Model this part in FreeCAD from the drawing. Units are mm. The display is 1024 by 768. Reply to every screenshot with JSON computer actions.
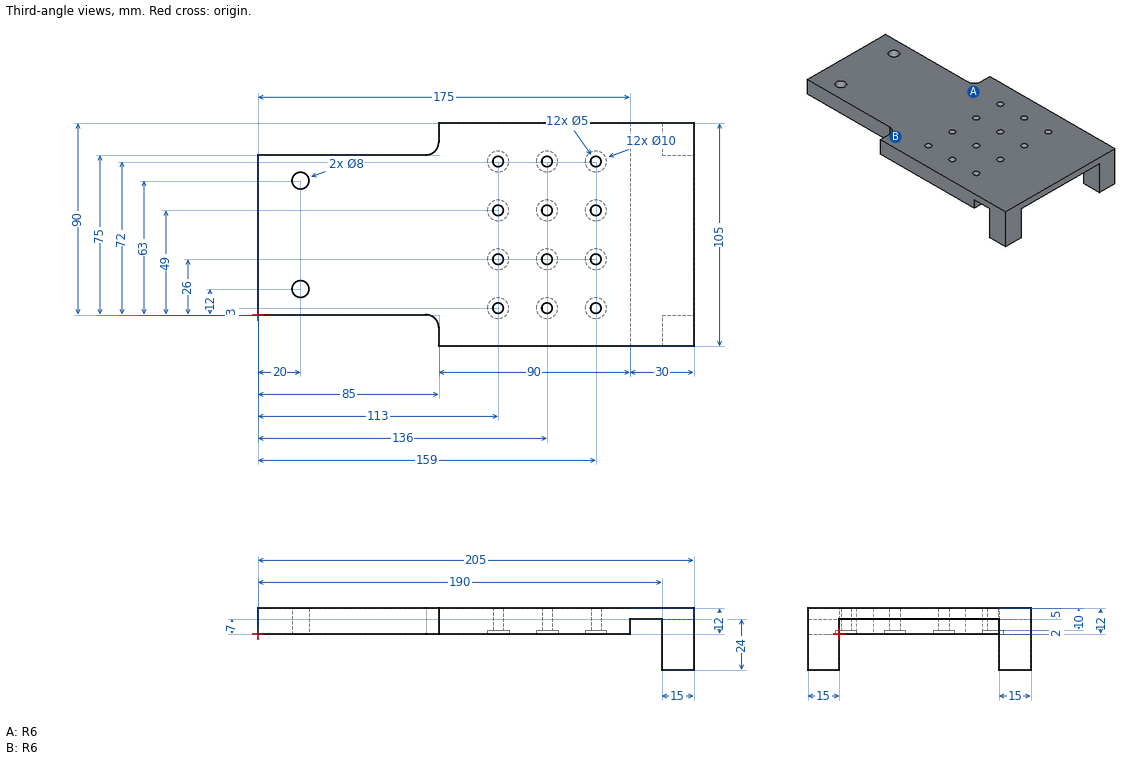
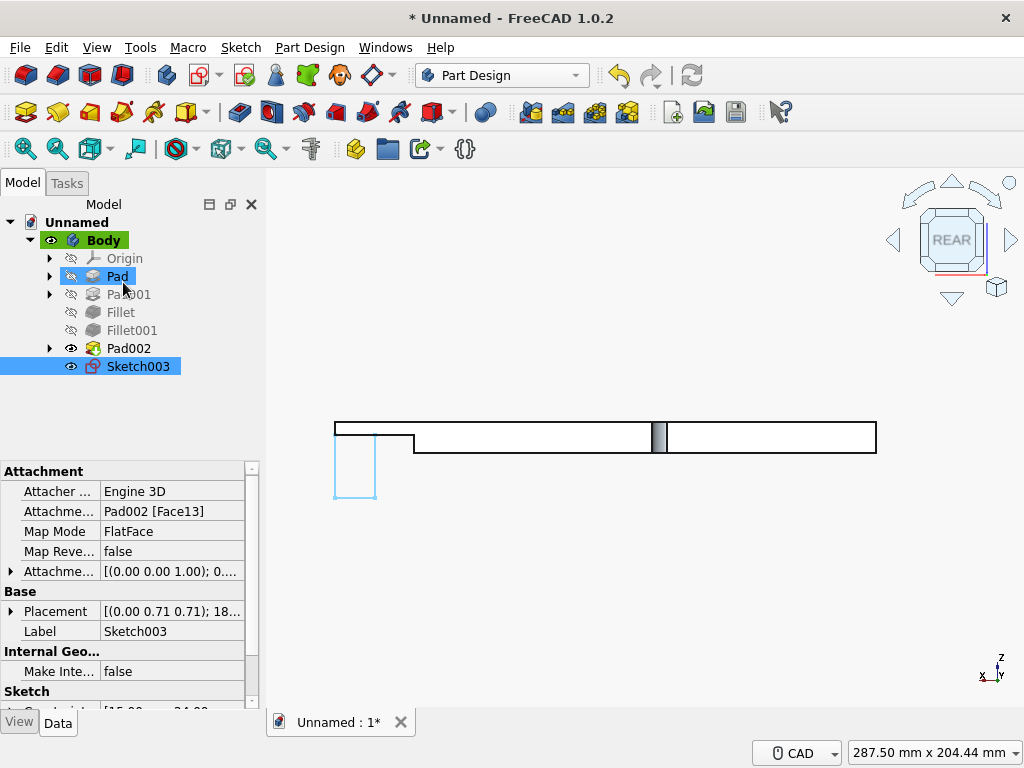
{"action": "left_click", "coordinate": [26, 112]}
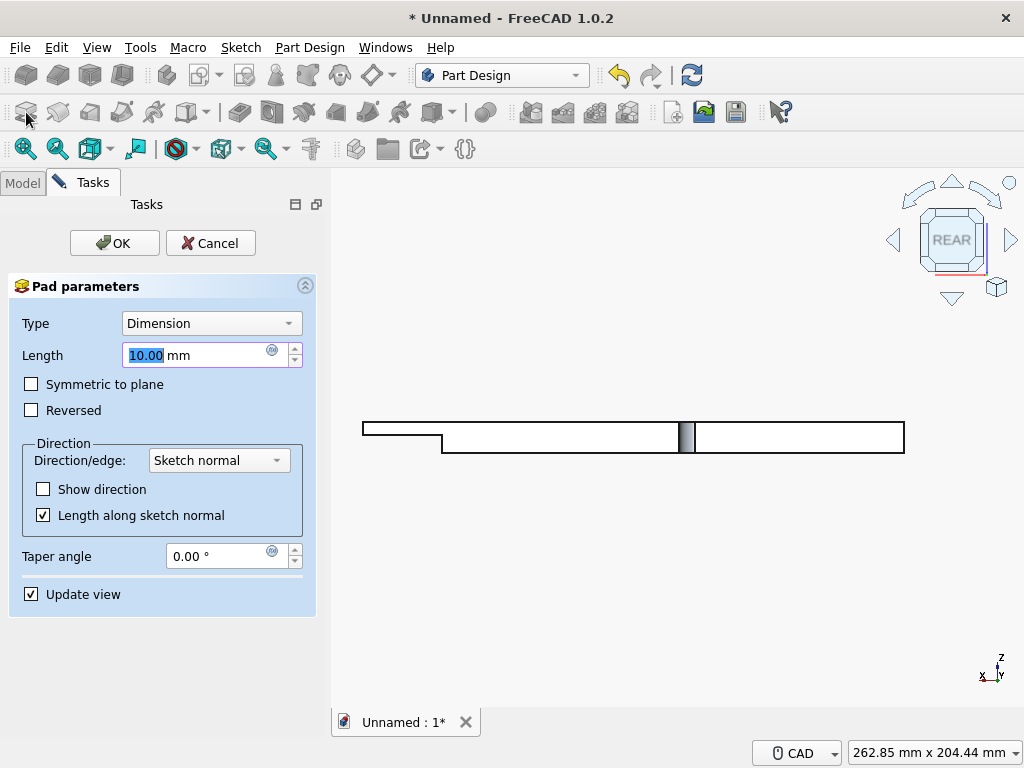
{"action": "type", "text": "15"}
{"action": "key", "text": "Tab"}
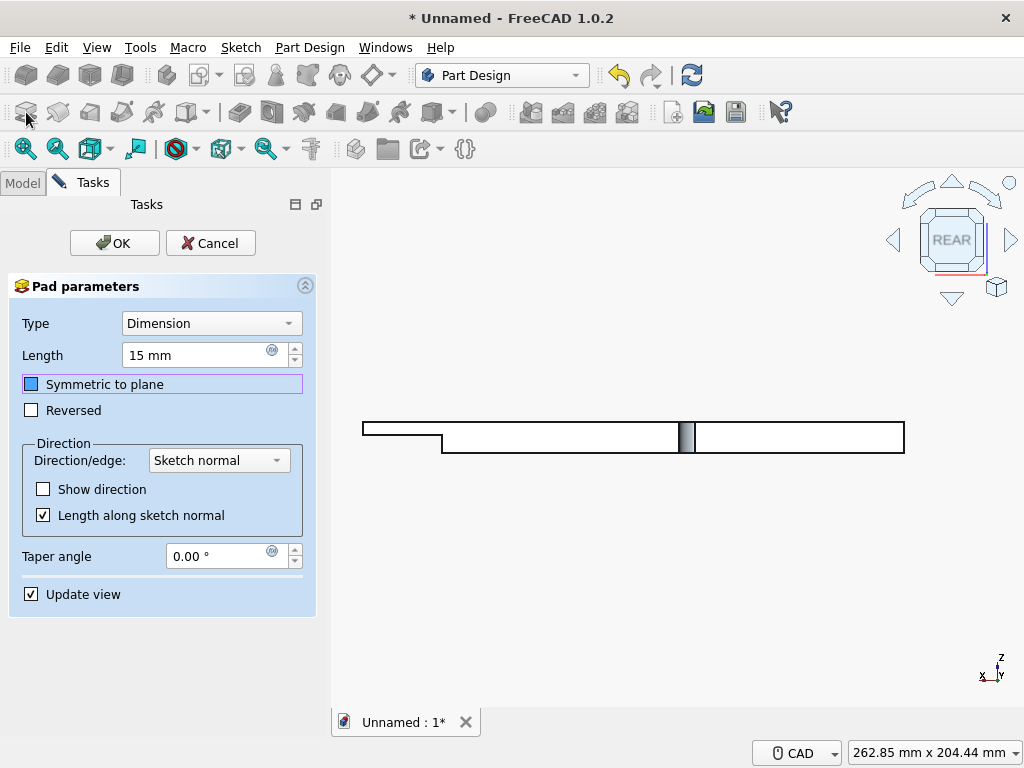
{"action": "left_click", "coordinate": [30, 410]}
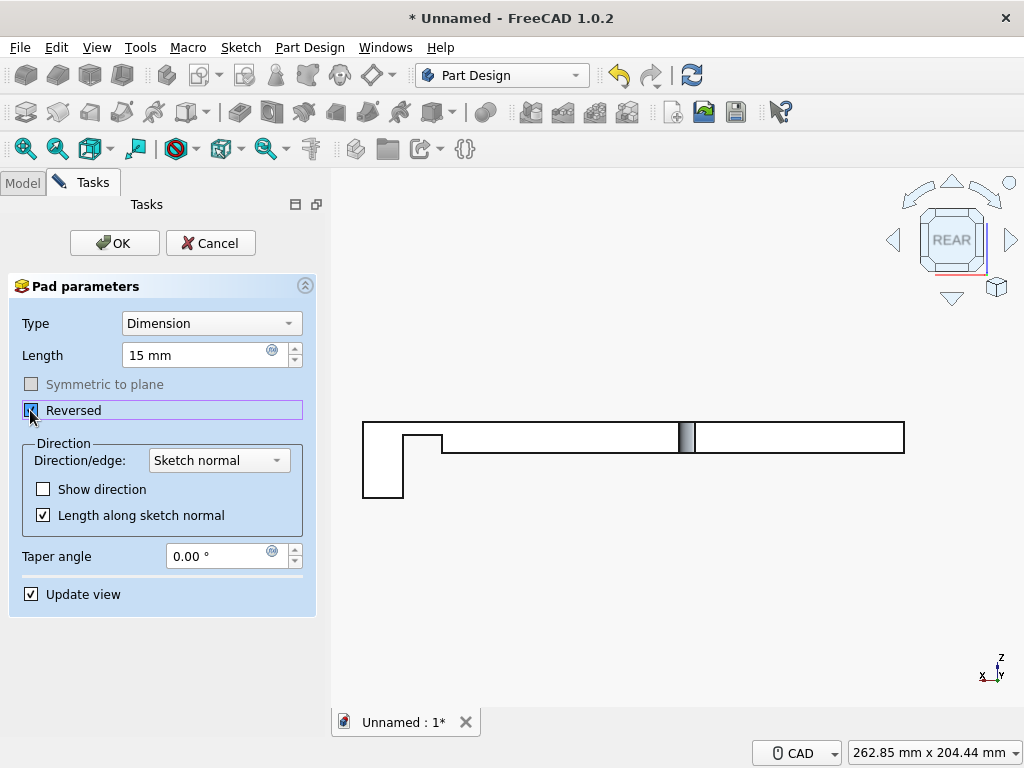
{"action": "left_click", "coordinate": [115, 243]}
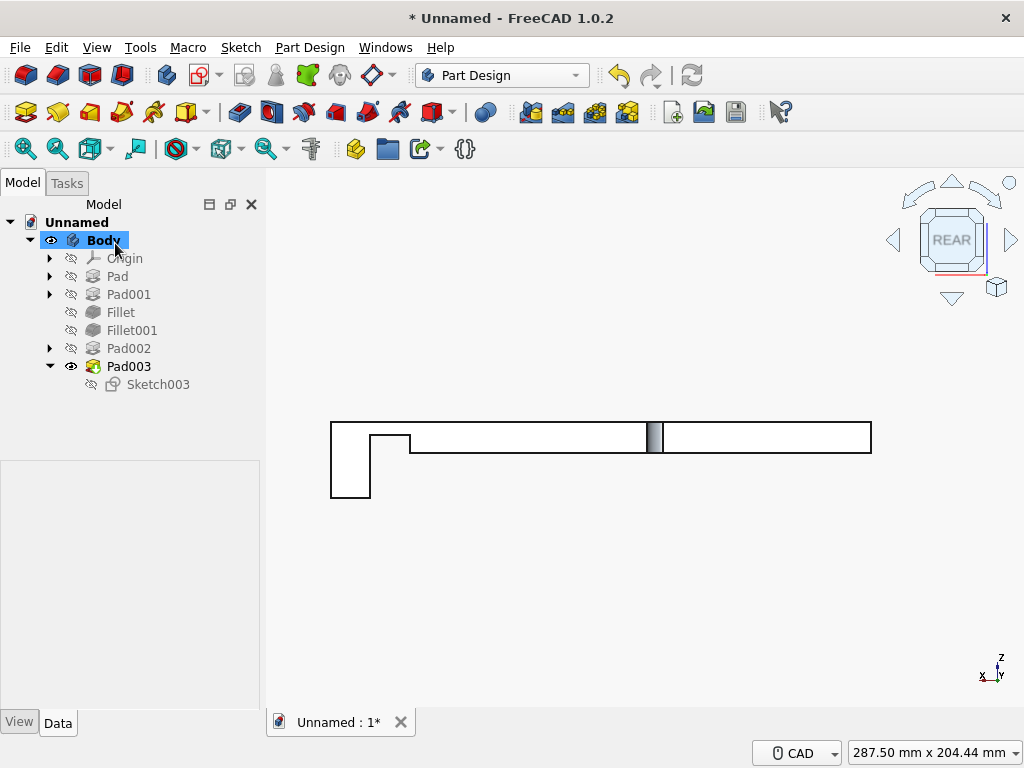
{"action": "key", "text": "0"}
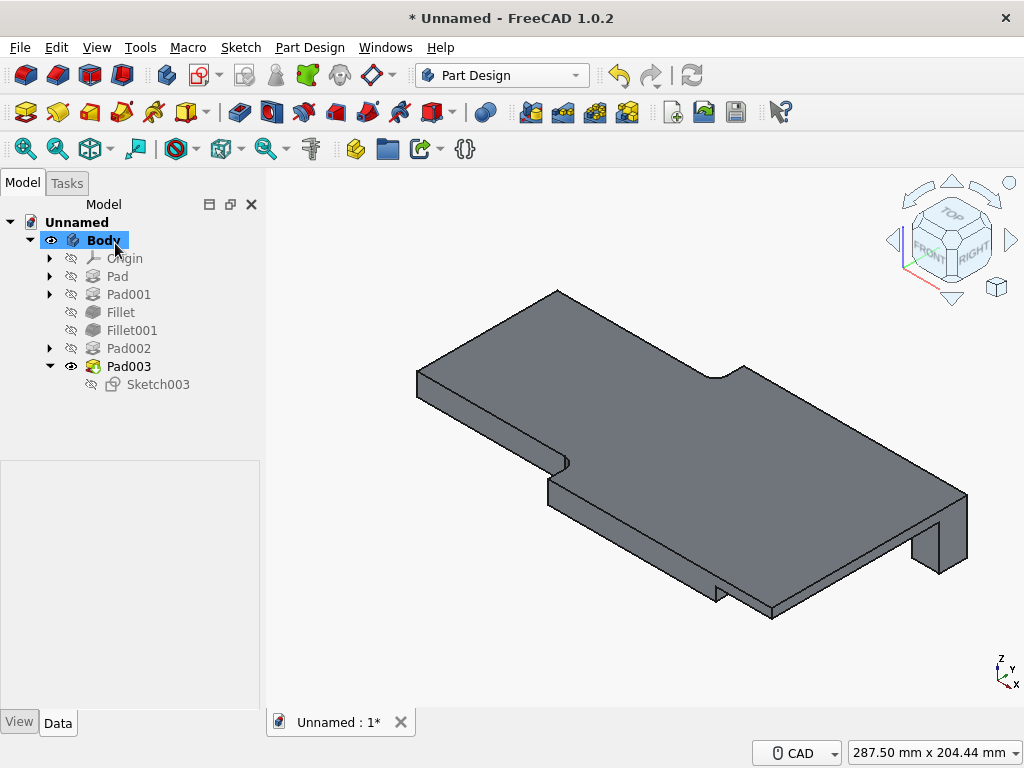
{"action": "left_click", "coordinate": [692, 574]}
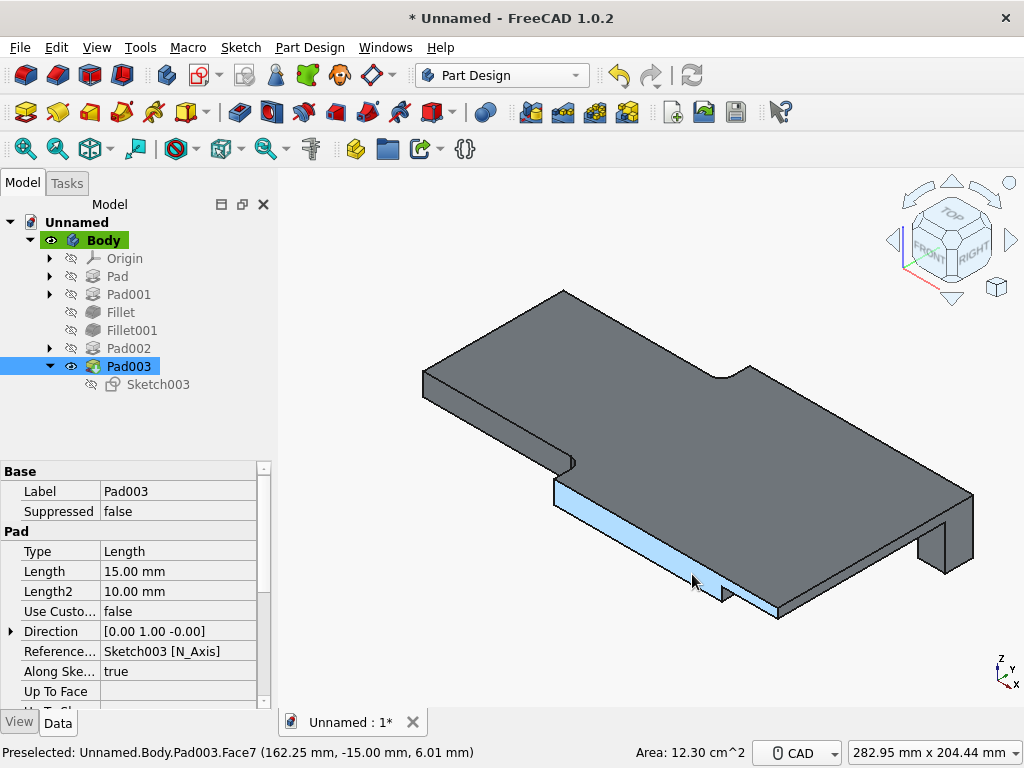
{"action": "left_click", "coordinate": [200, 76]}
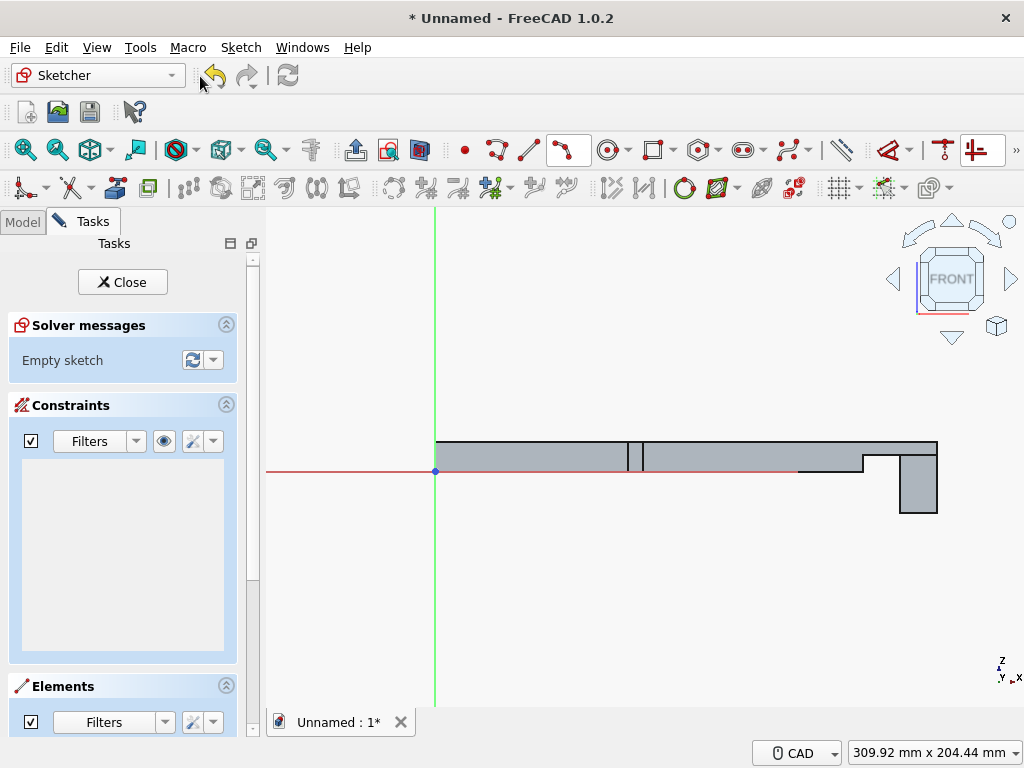
{"action": "scroll", "coordinate": [576, 457], "scroll_direction": "down", "scroll_amount": 5}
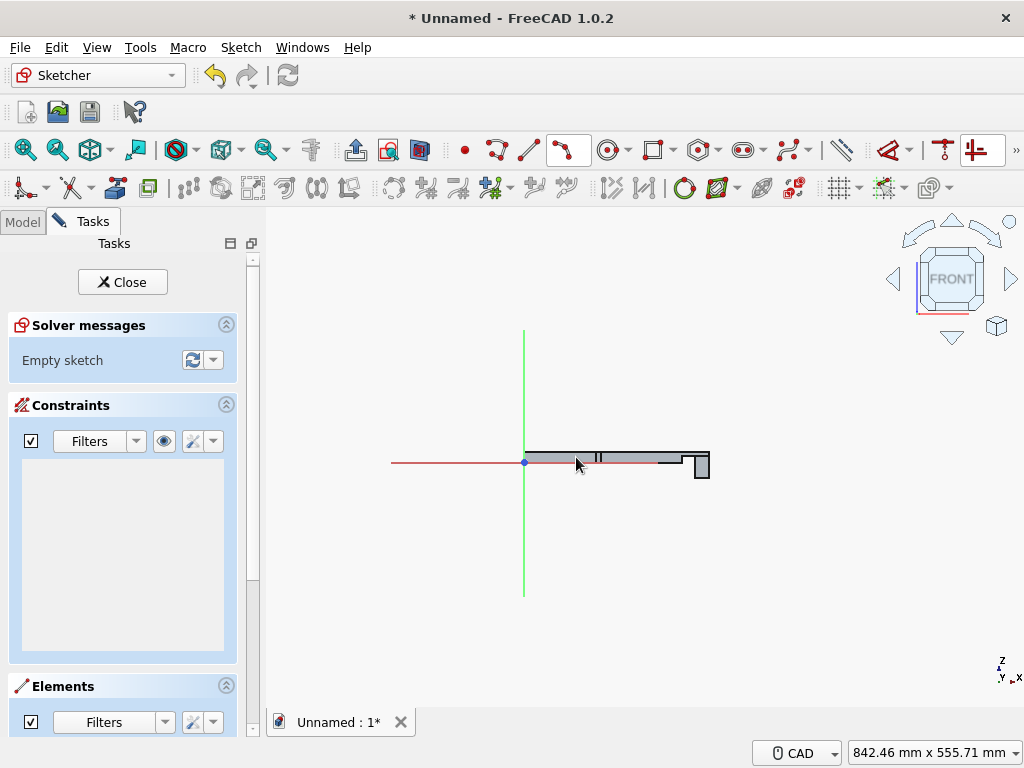
{"action": "scroll", "coordinate": [712, 468], "scroll_direction": "up", "scroll_amount": 13}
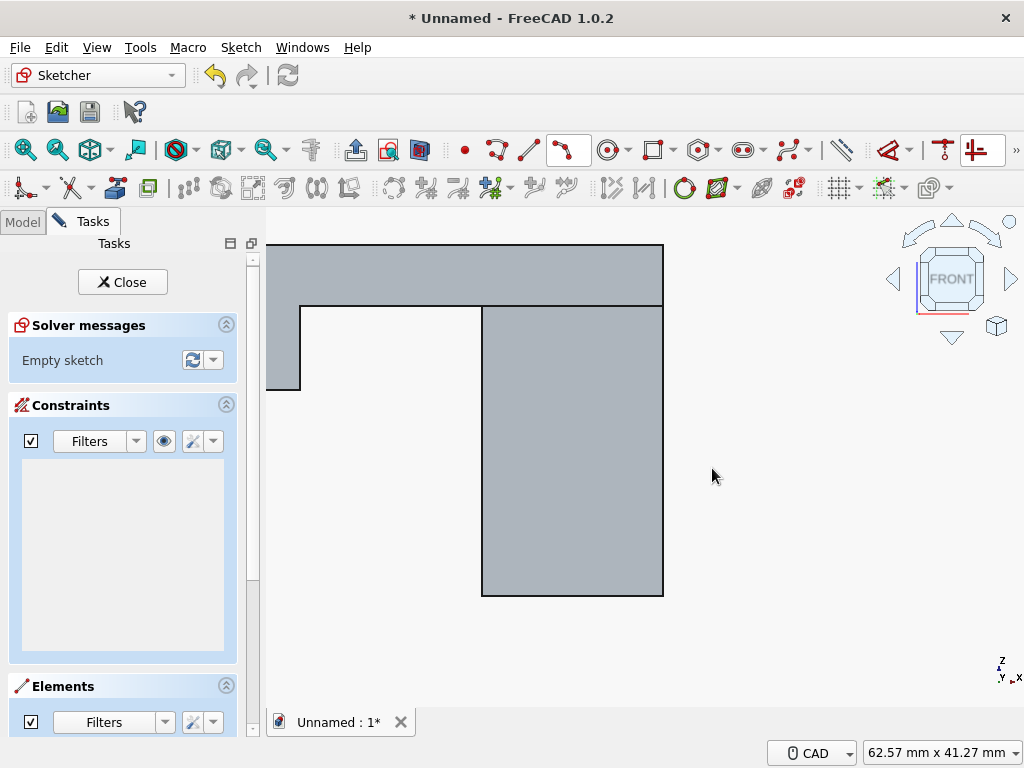
{"action": "left_click", "coordinate": [654, 150]}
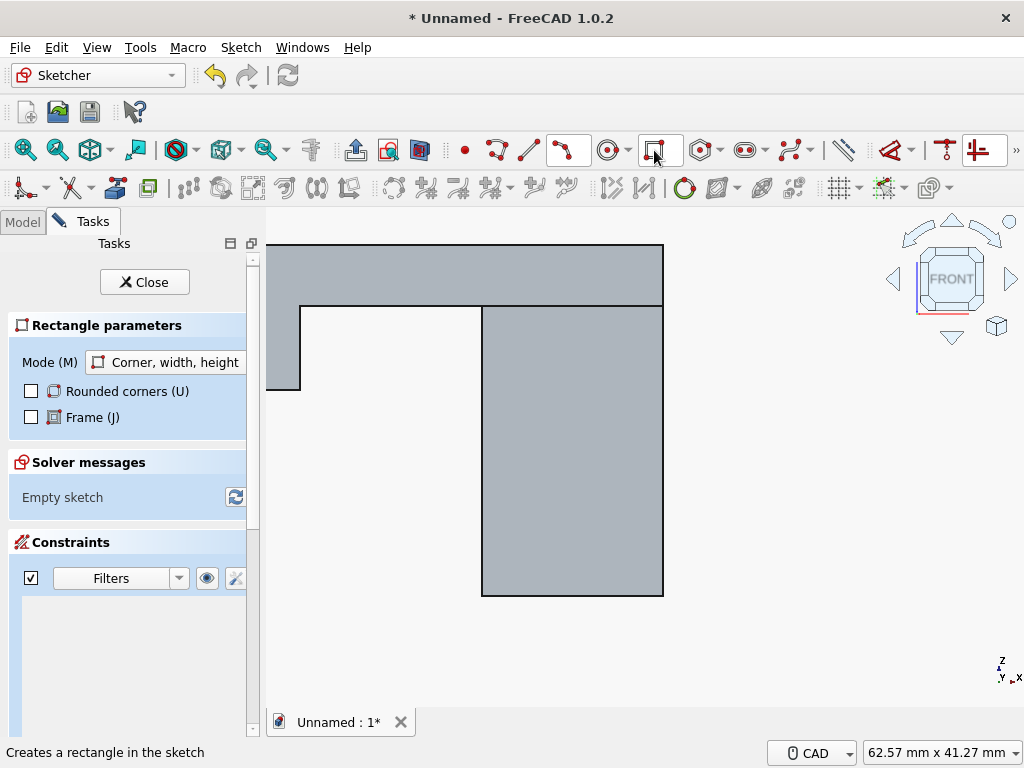
{"action": "left_click", "coordinate": [482, 306]}
{"action": "mouse_move", "coordinate": [663, 596]}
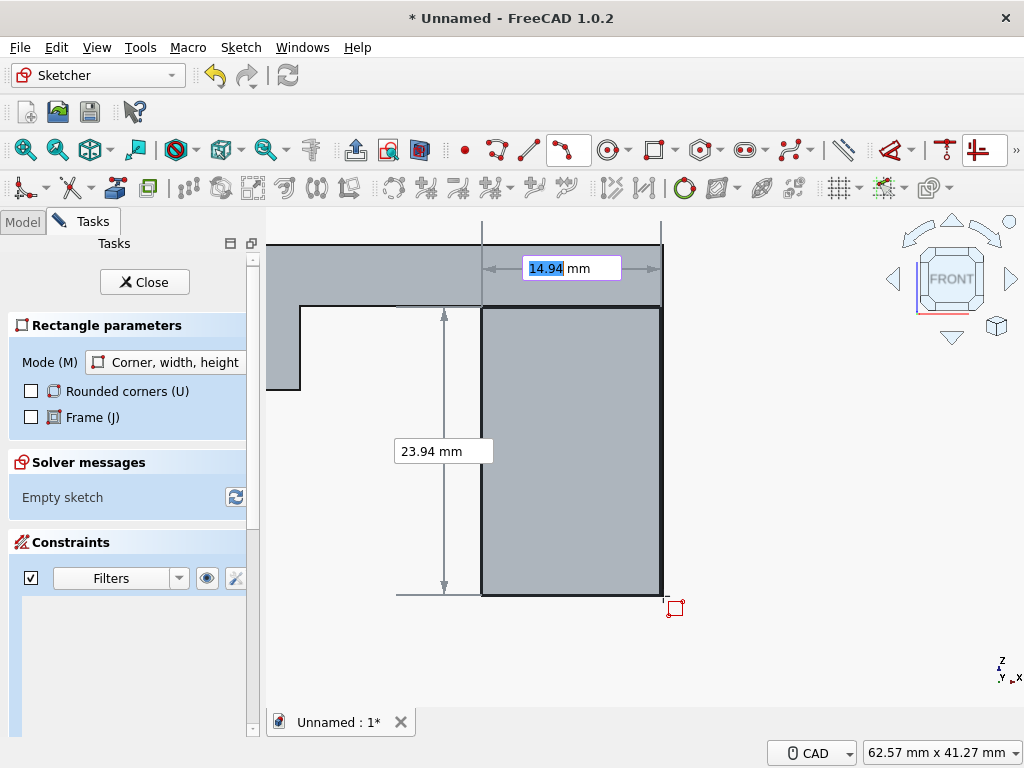
{"action": "type", "text": "15"}
{"action": "key", "text": "Tab"}
{"action": "type", "text": "24"}
{"action": "key", "text": "Return"}
{"action": "key", "text": "Escape"}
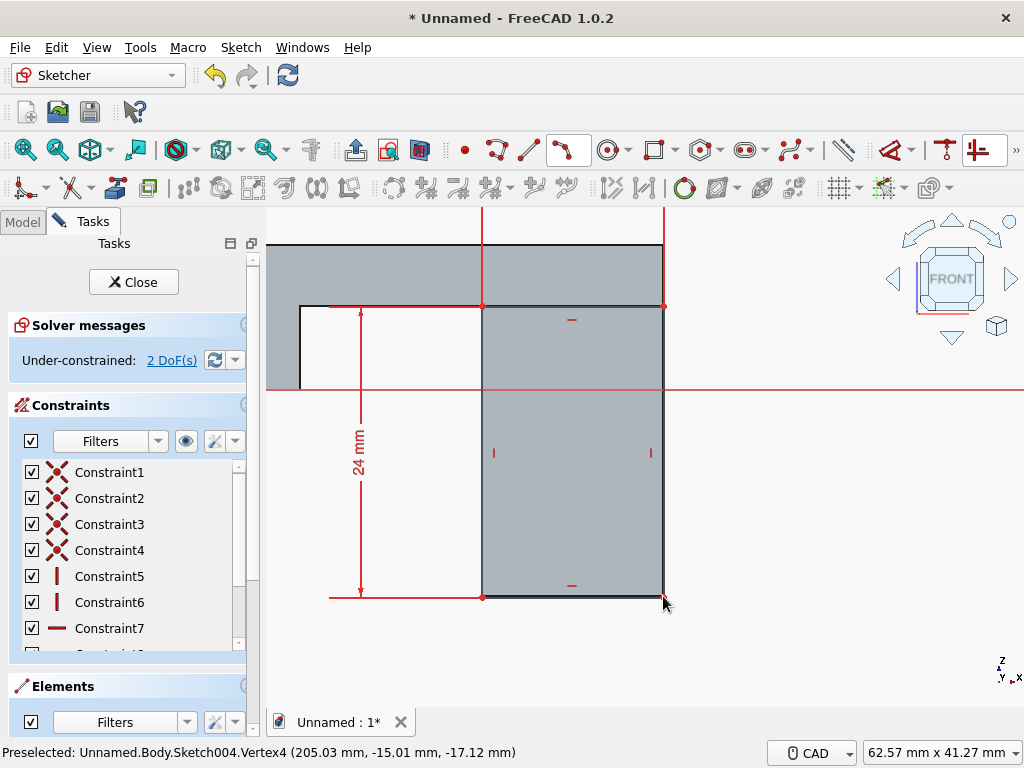
{"action": "left_click", "coordinate": [890, 150]}